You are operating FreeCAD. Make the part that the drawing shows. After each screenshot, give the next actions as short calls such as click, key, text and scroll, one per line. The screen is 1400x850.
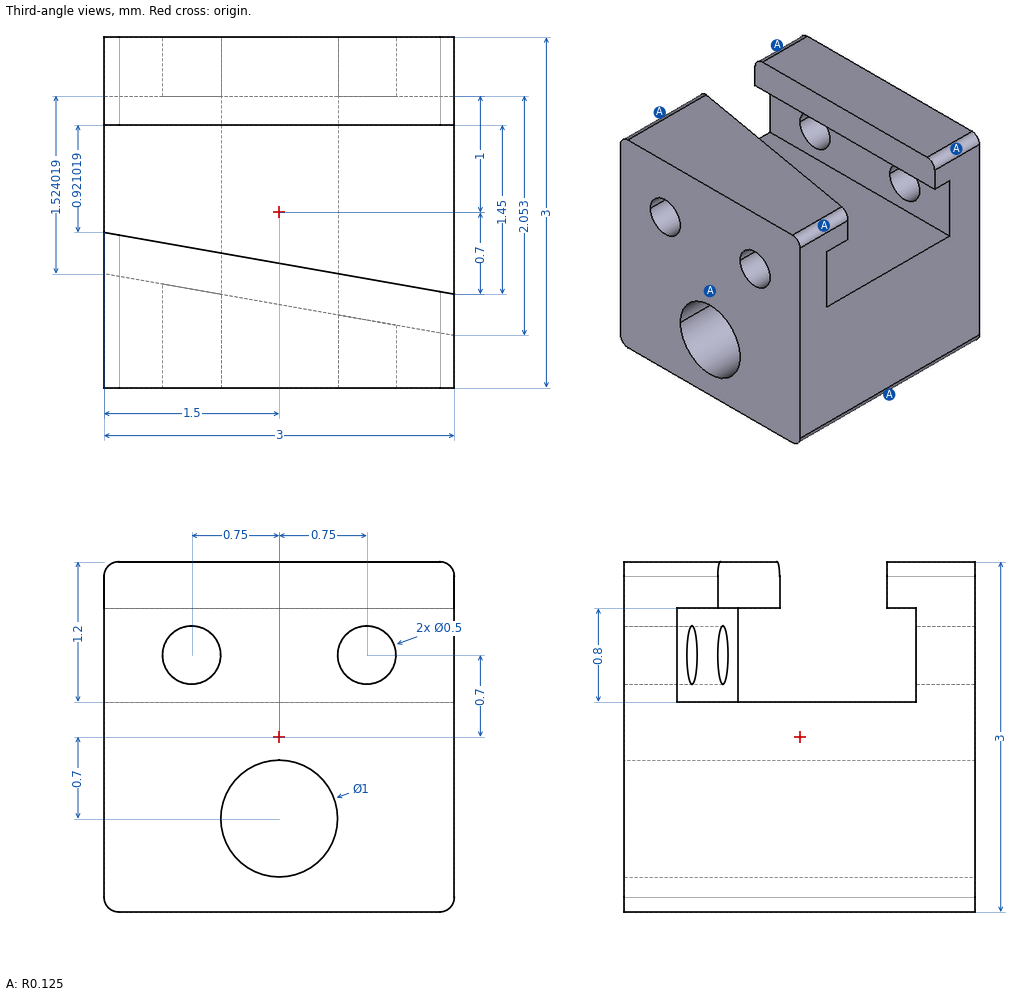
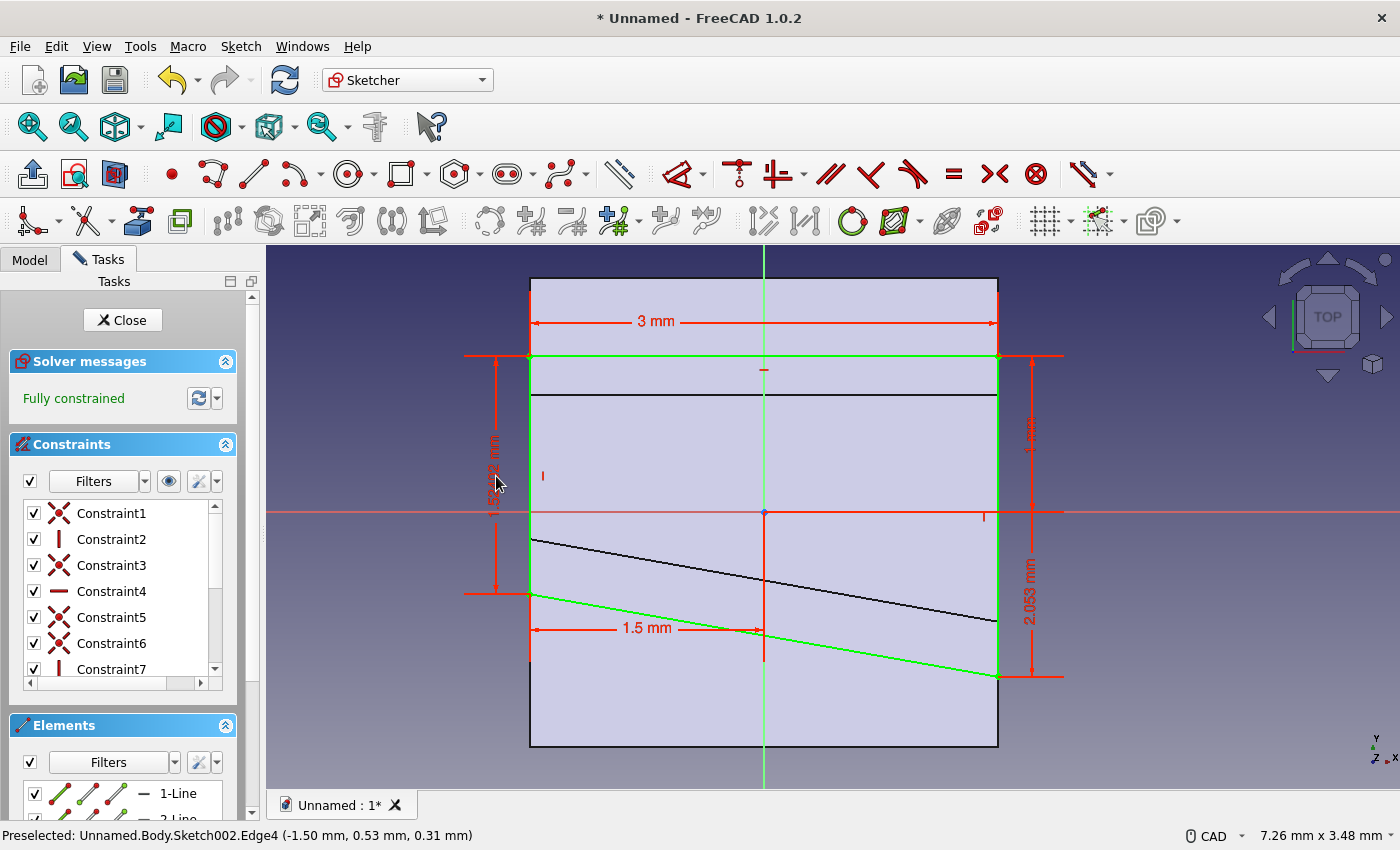
click(123, 320)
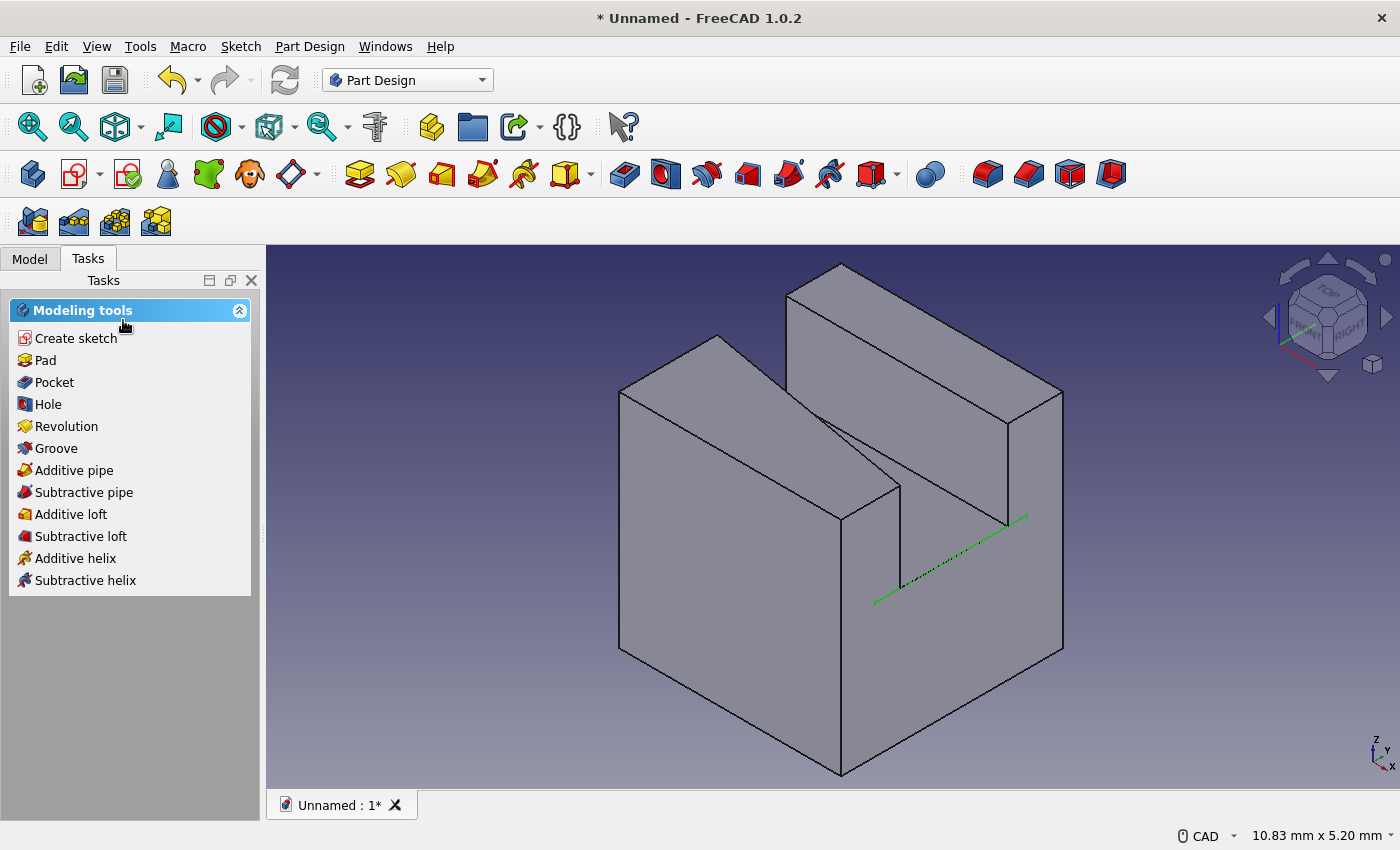
click(625, 174)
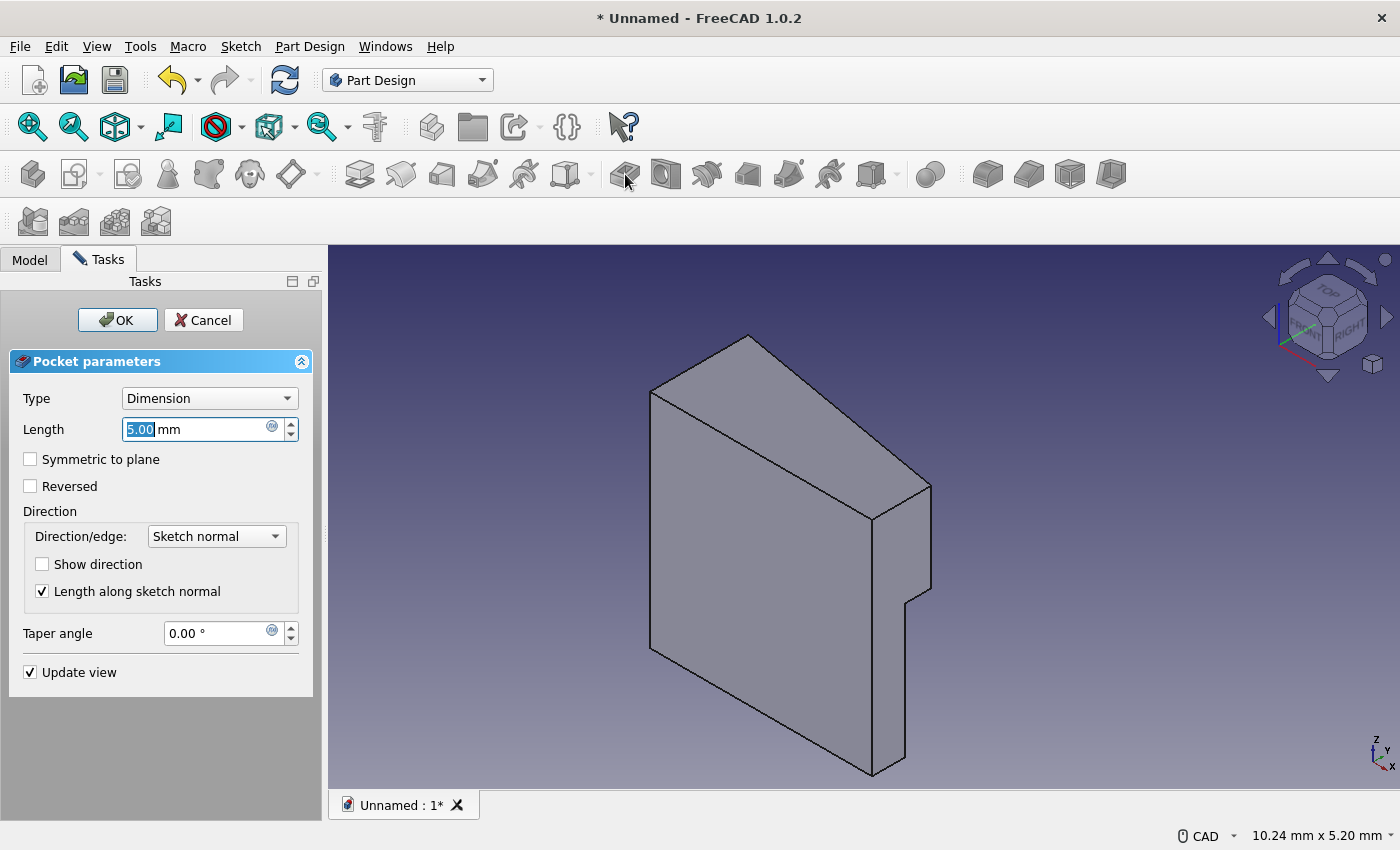
text(0.8)
key(Tab)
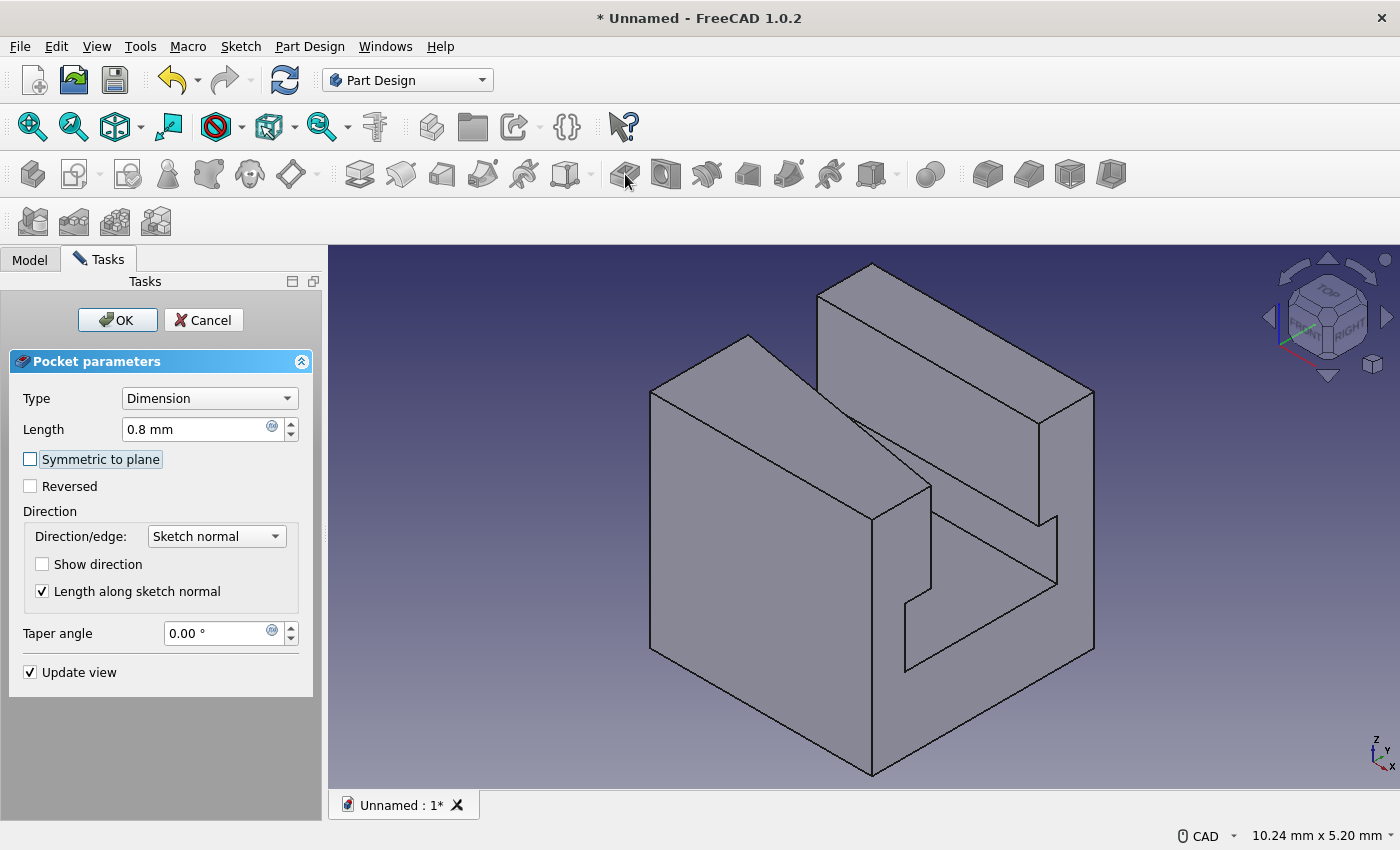
click(31, 486)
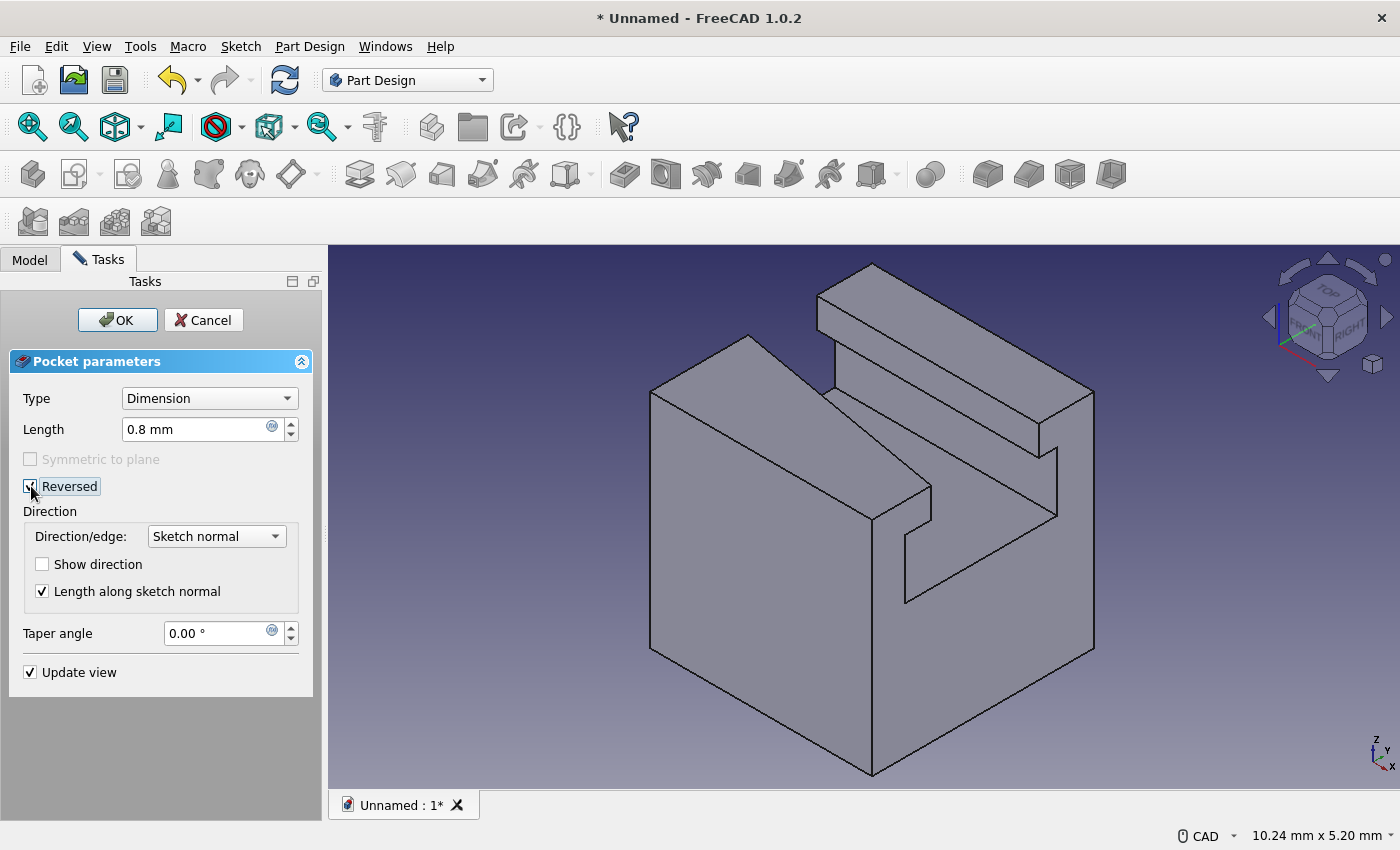
click(118, 320)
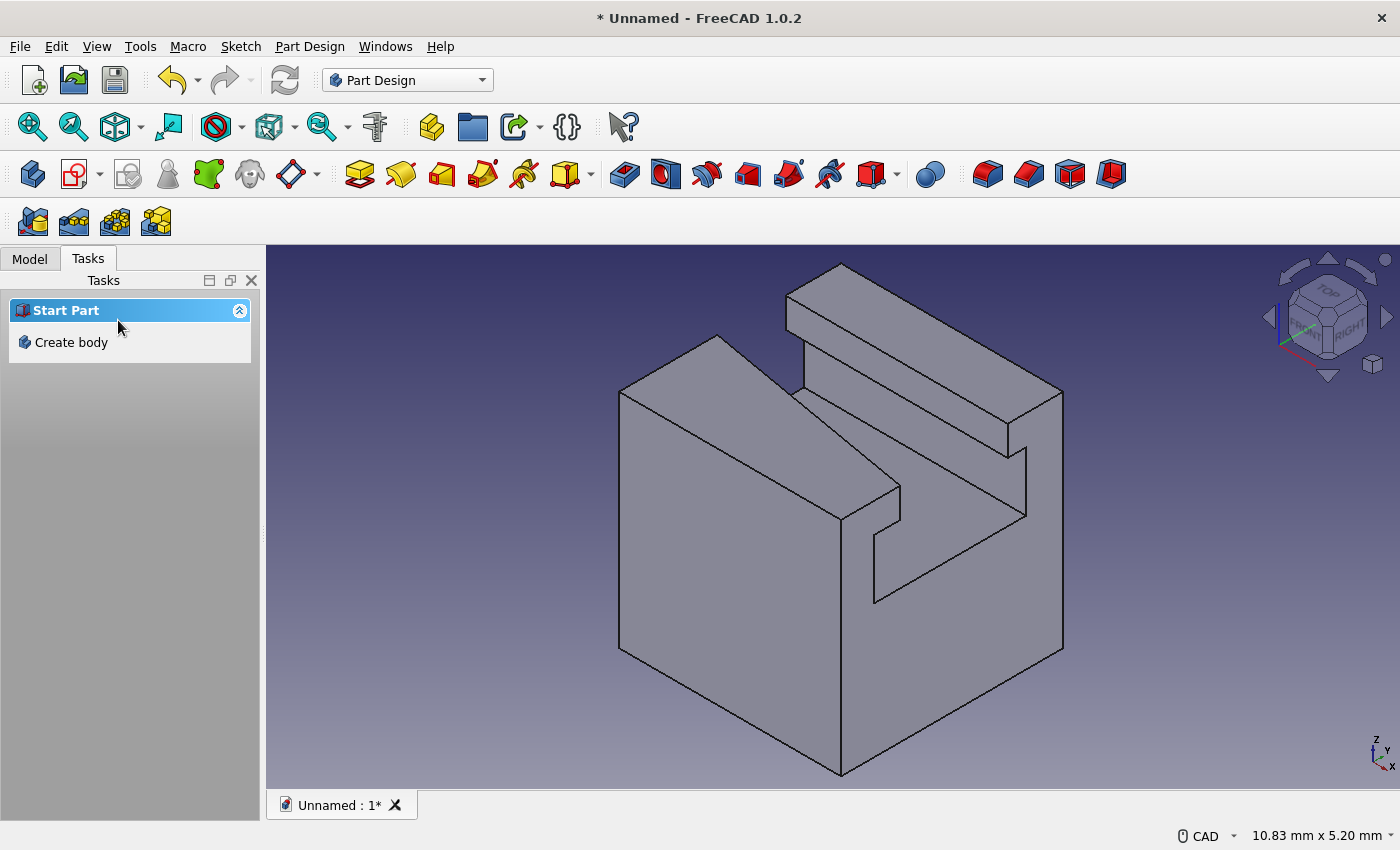
click(1035, 407)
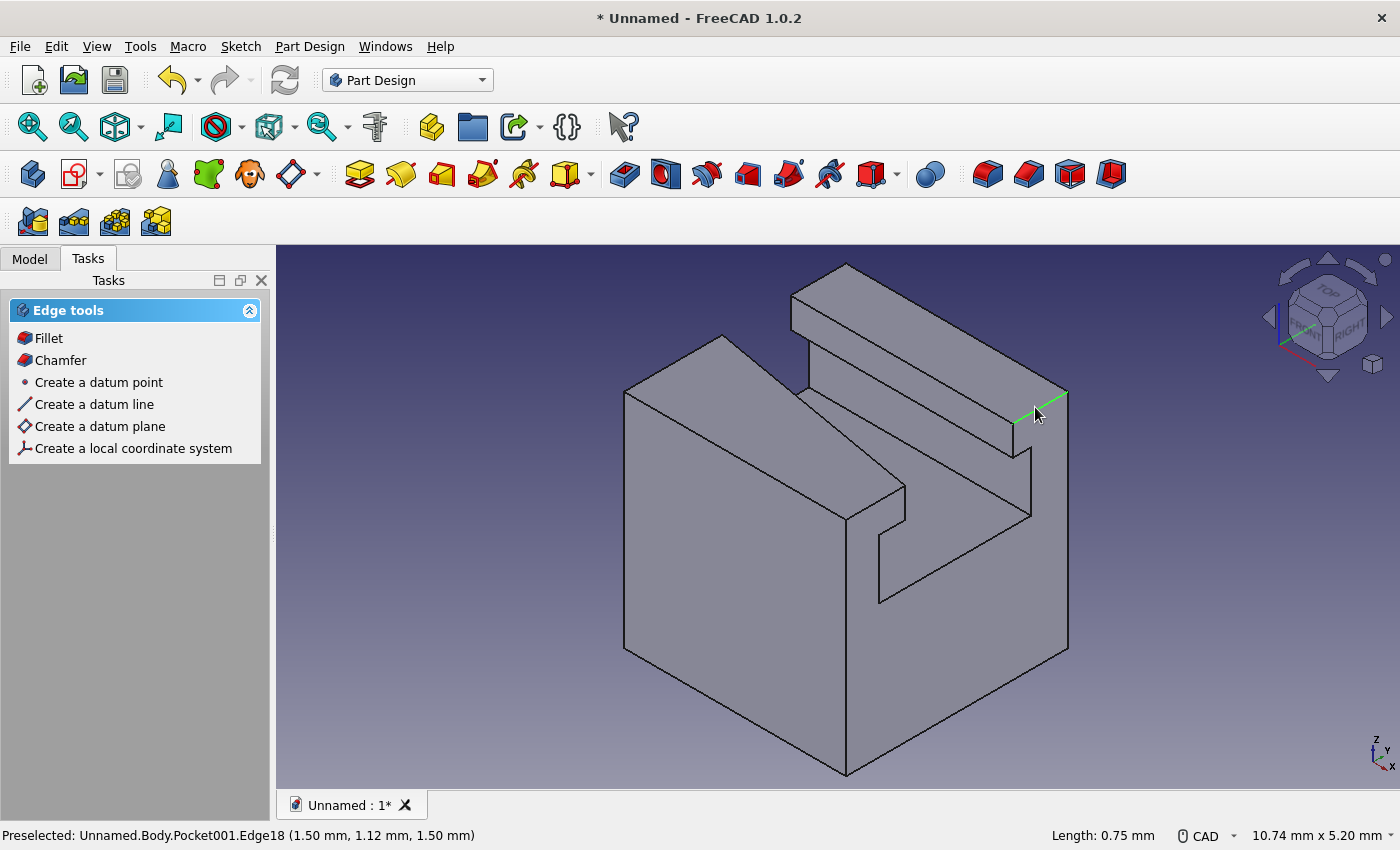
click(876, 502, ctrl)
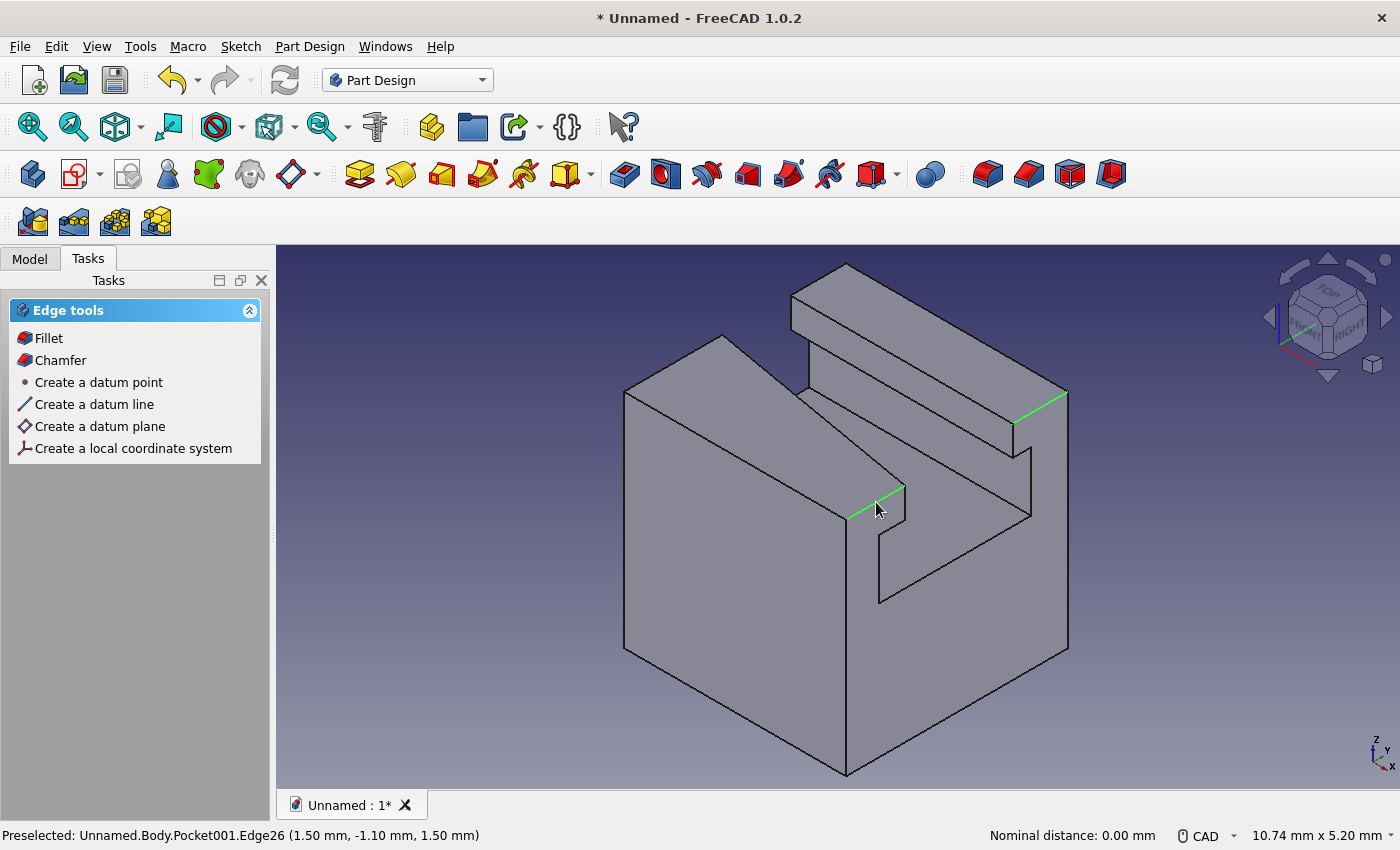
key(2)